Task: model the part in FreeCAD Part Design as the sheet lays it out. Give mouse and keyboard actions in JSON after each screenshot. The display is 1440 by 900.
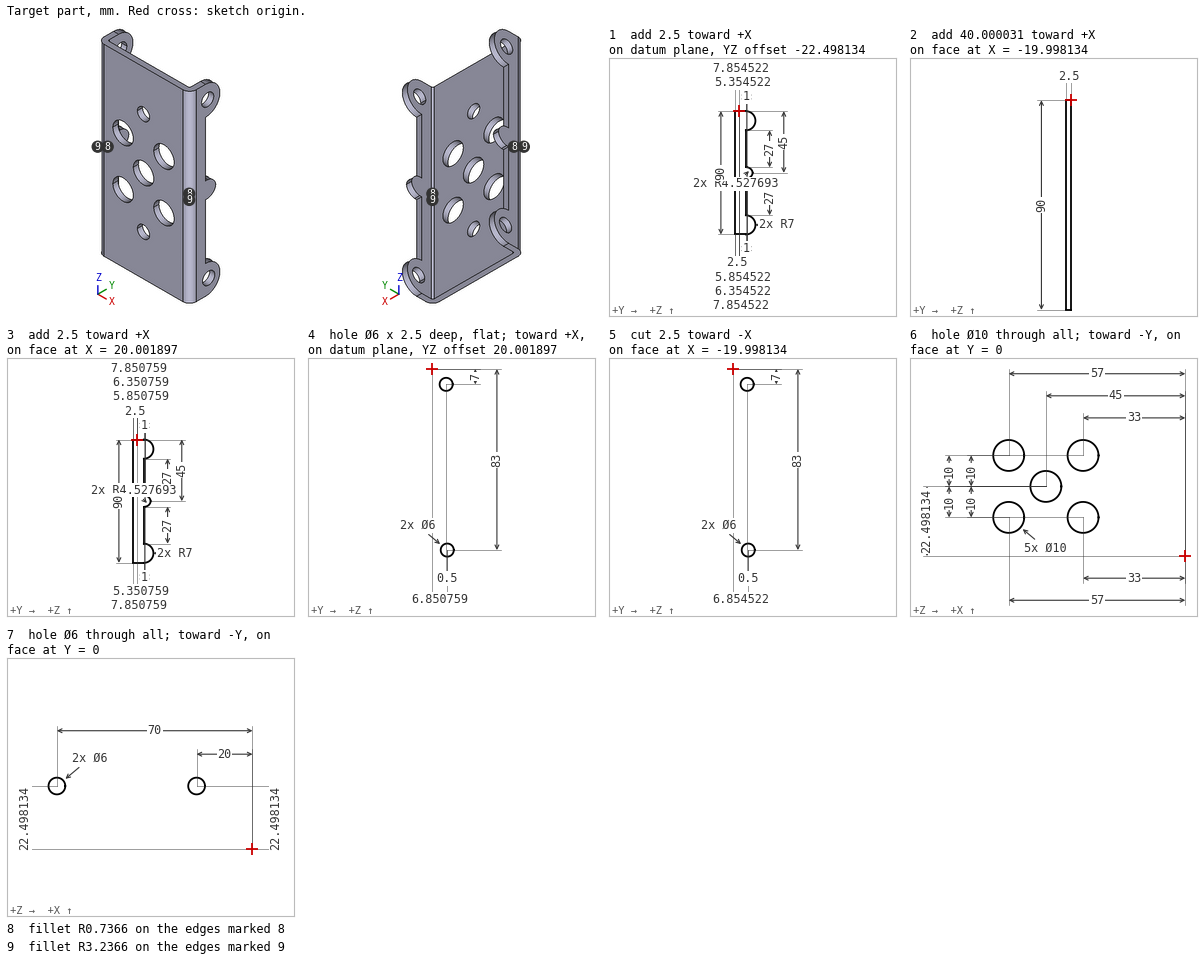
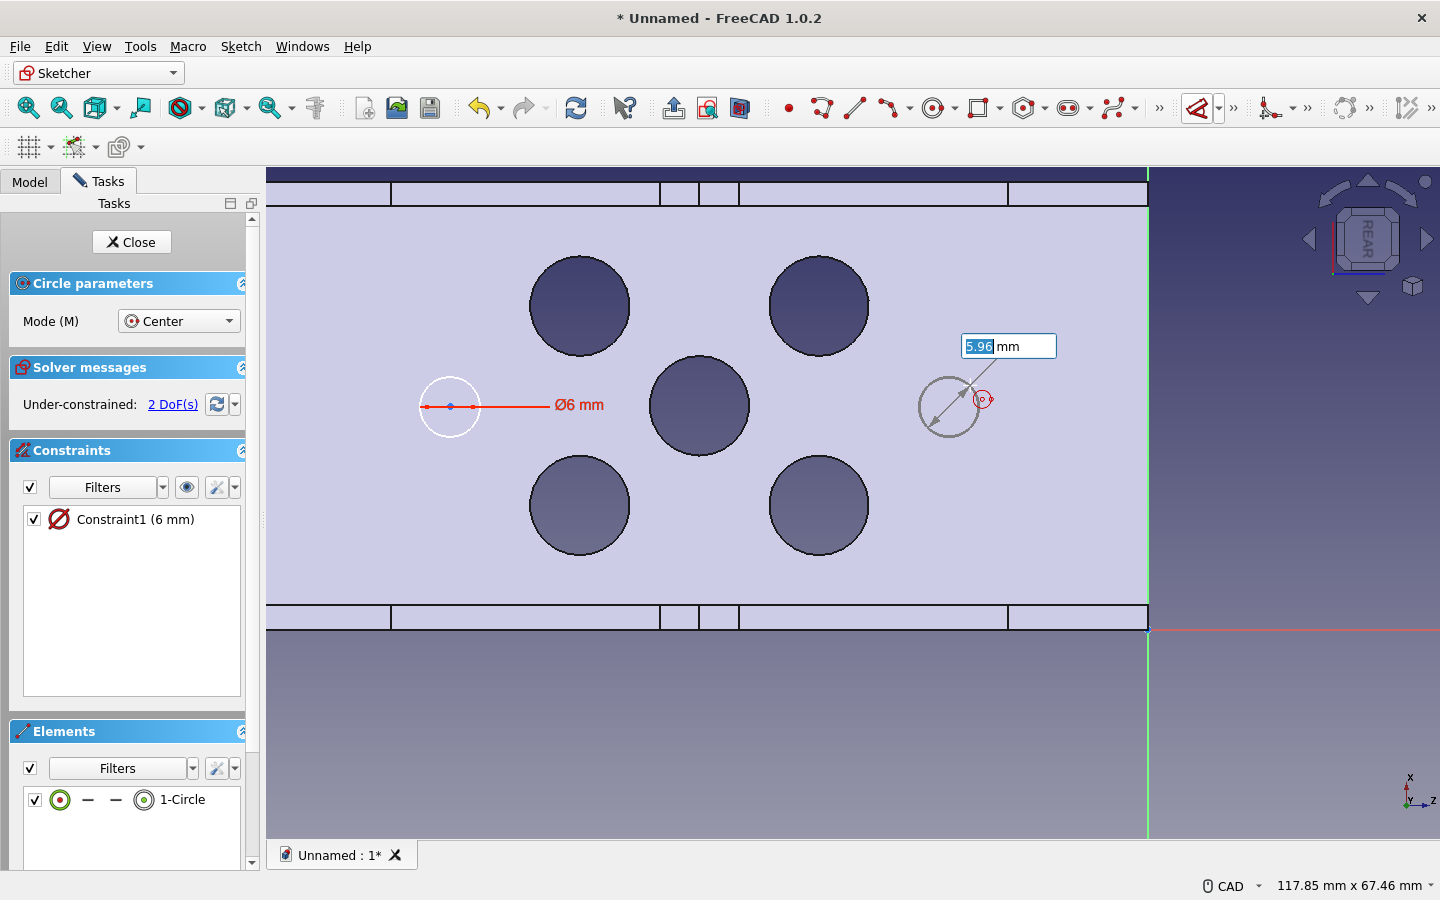
{"action": "type", "text": "6"}
{"action": "key", "text": "Return"}
{"action": "key", "text": "Escape"}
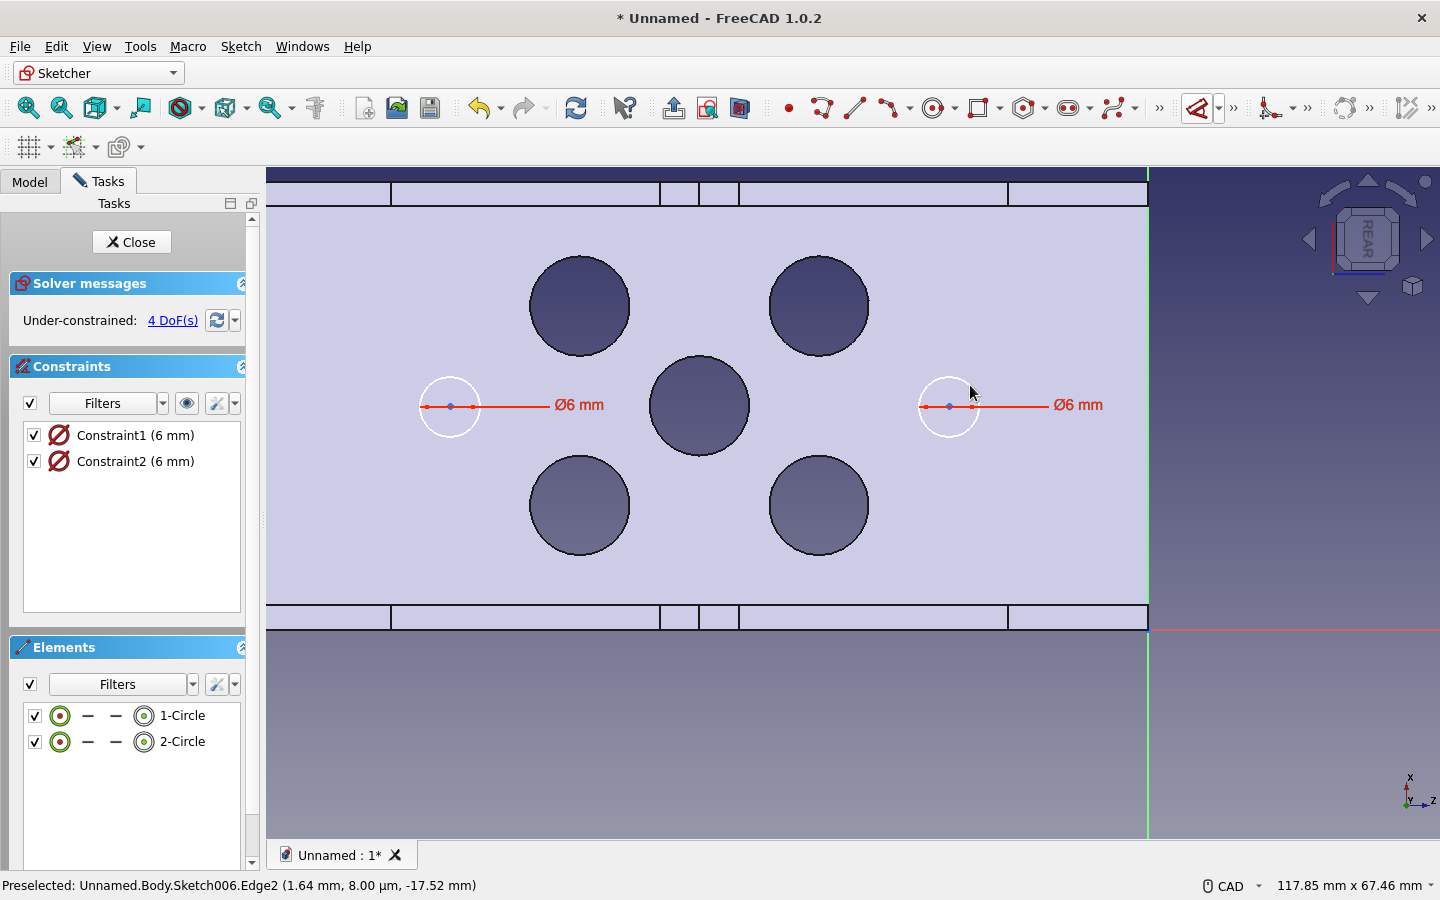
{"action": "left_click", "coordinate": [450, 407]}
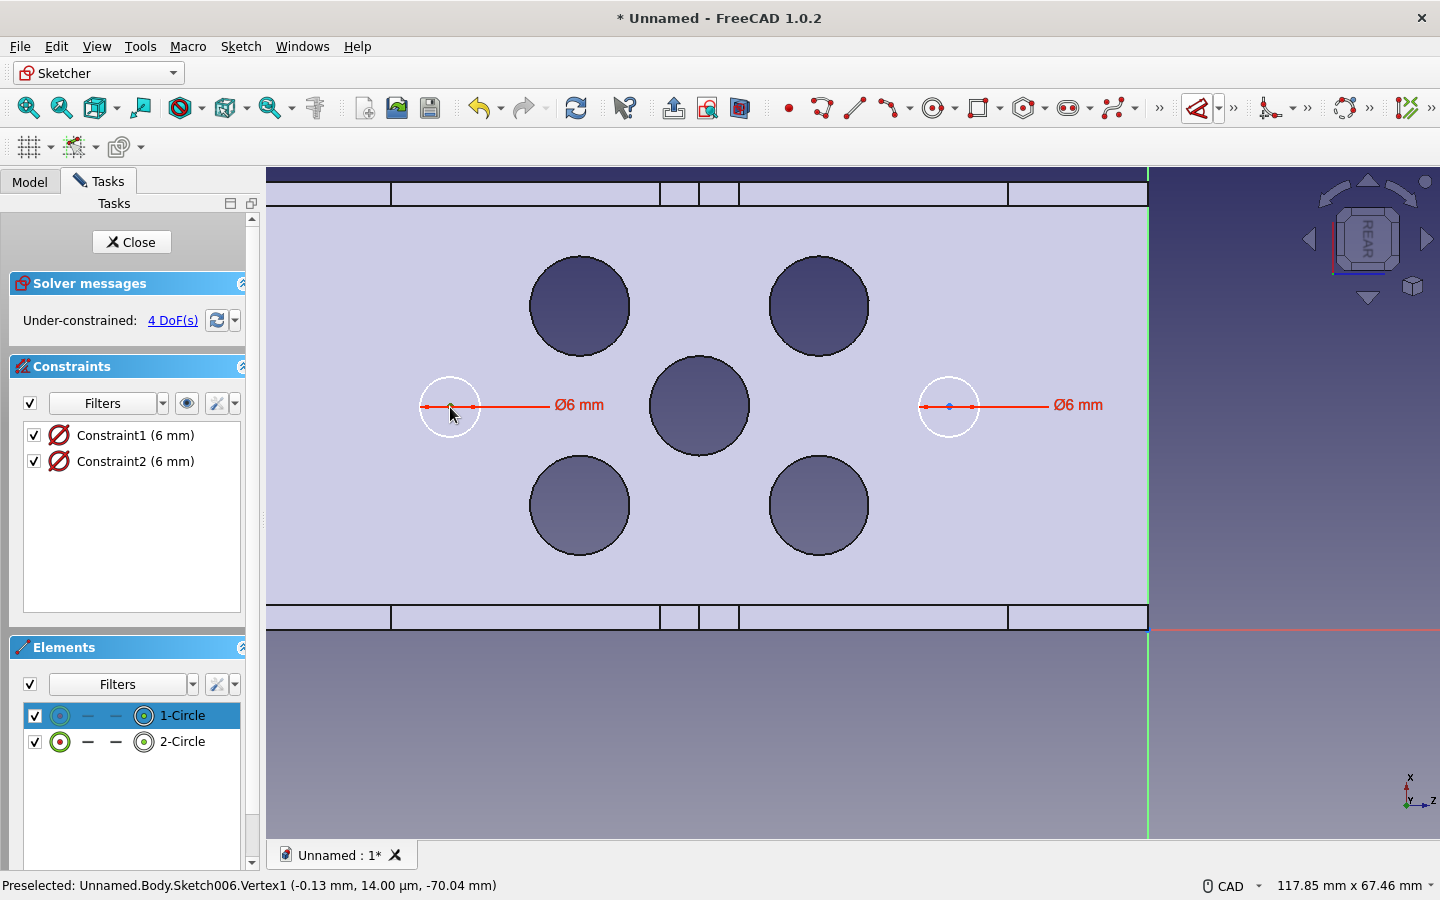
{"action": "left_click", "coordinate": [1218, 108]}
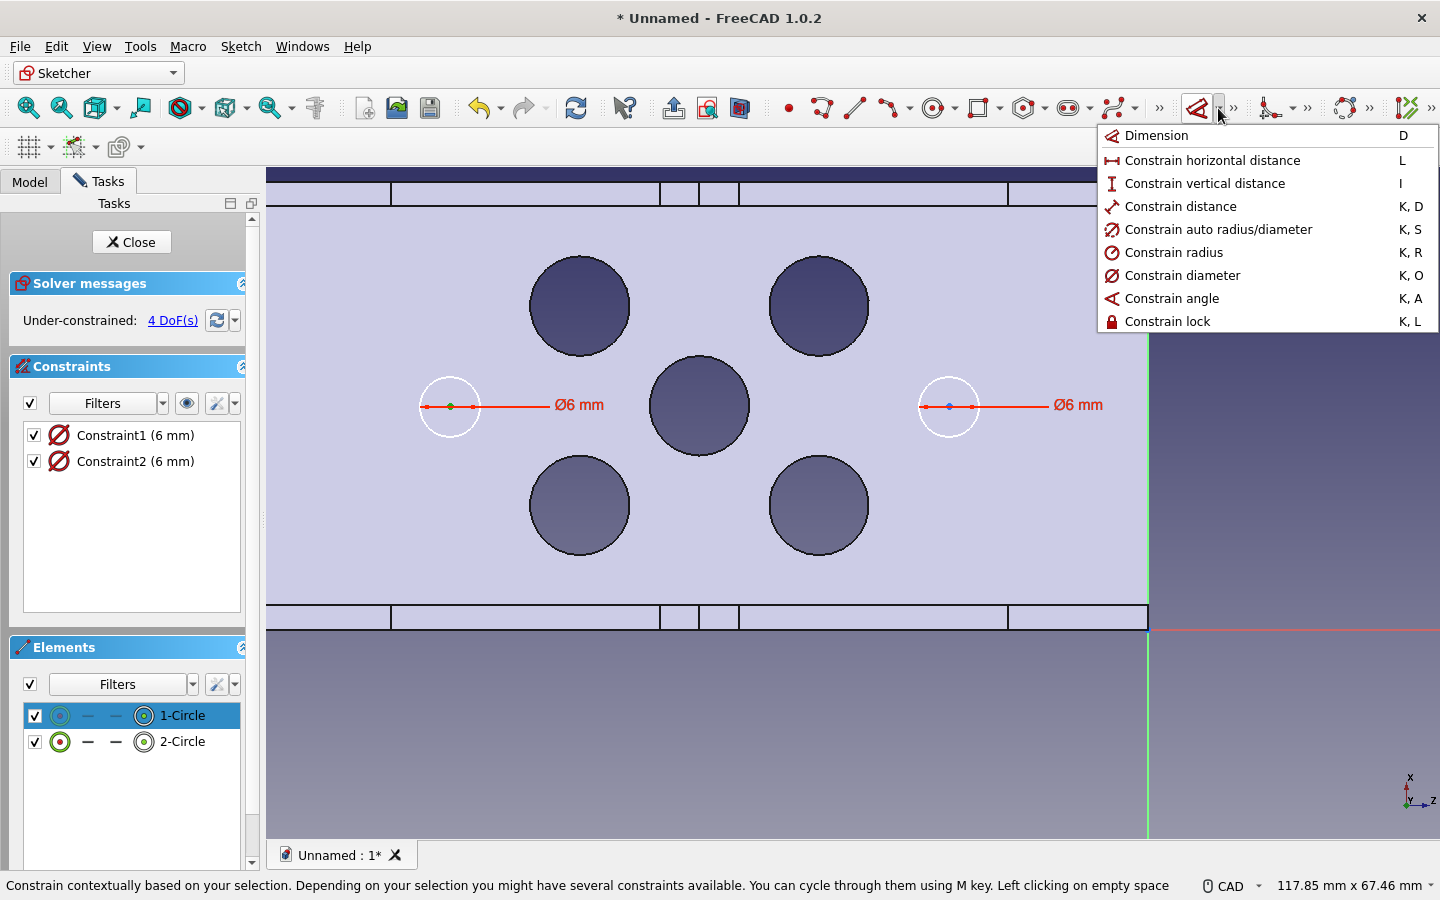
{"action": "left_click", "coordinate": [1268, 160]}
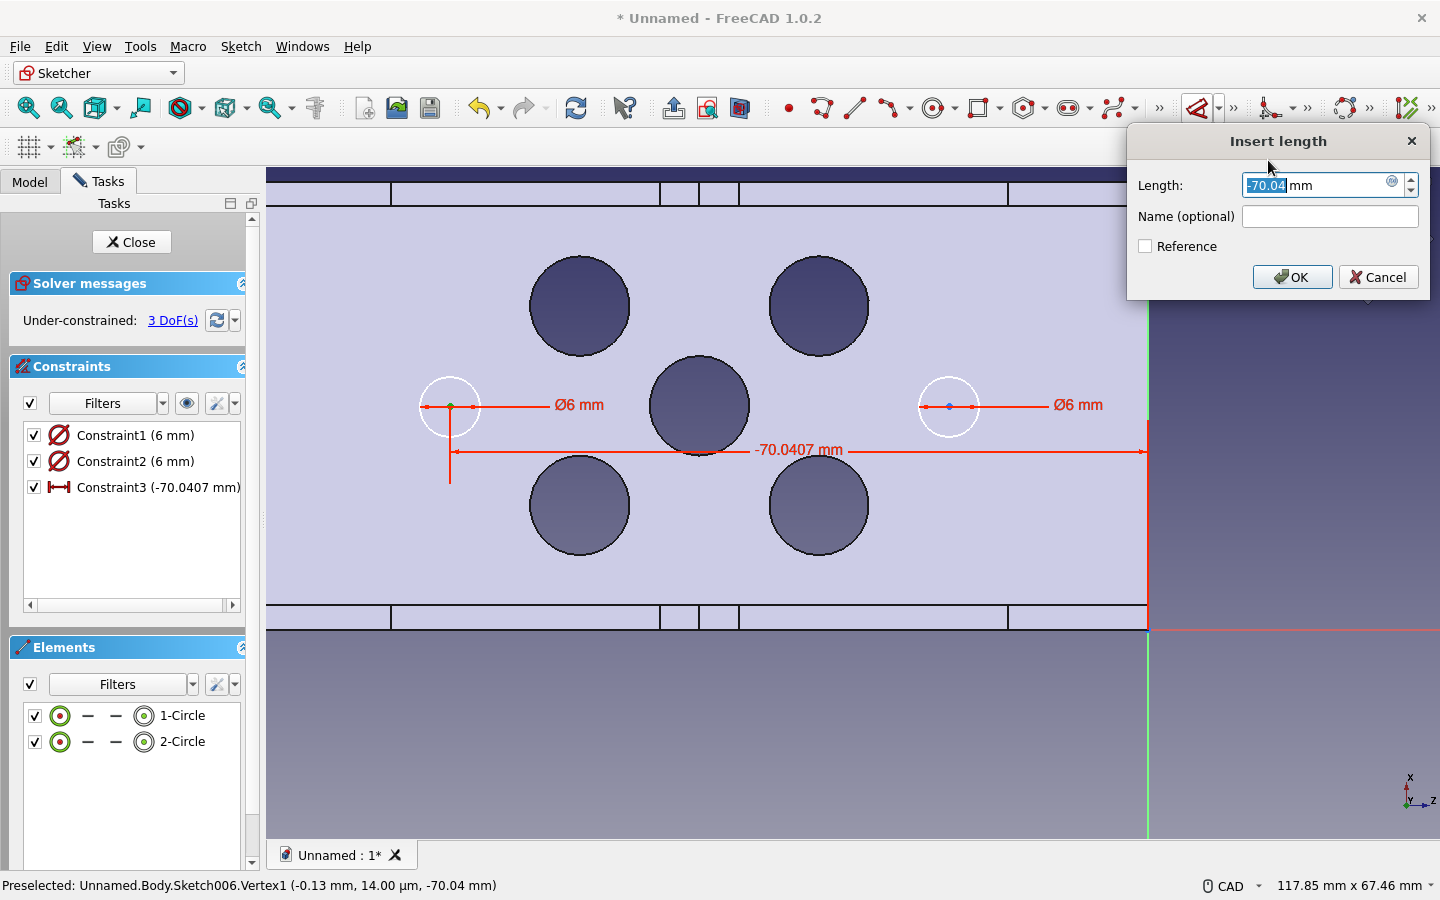
{"action": "type", "text": "-70"}
{"action": "key", "text": "Return"}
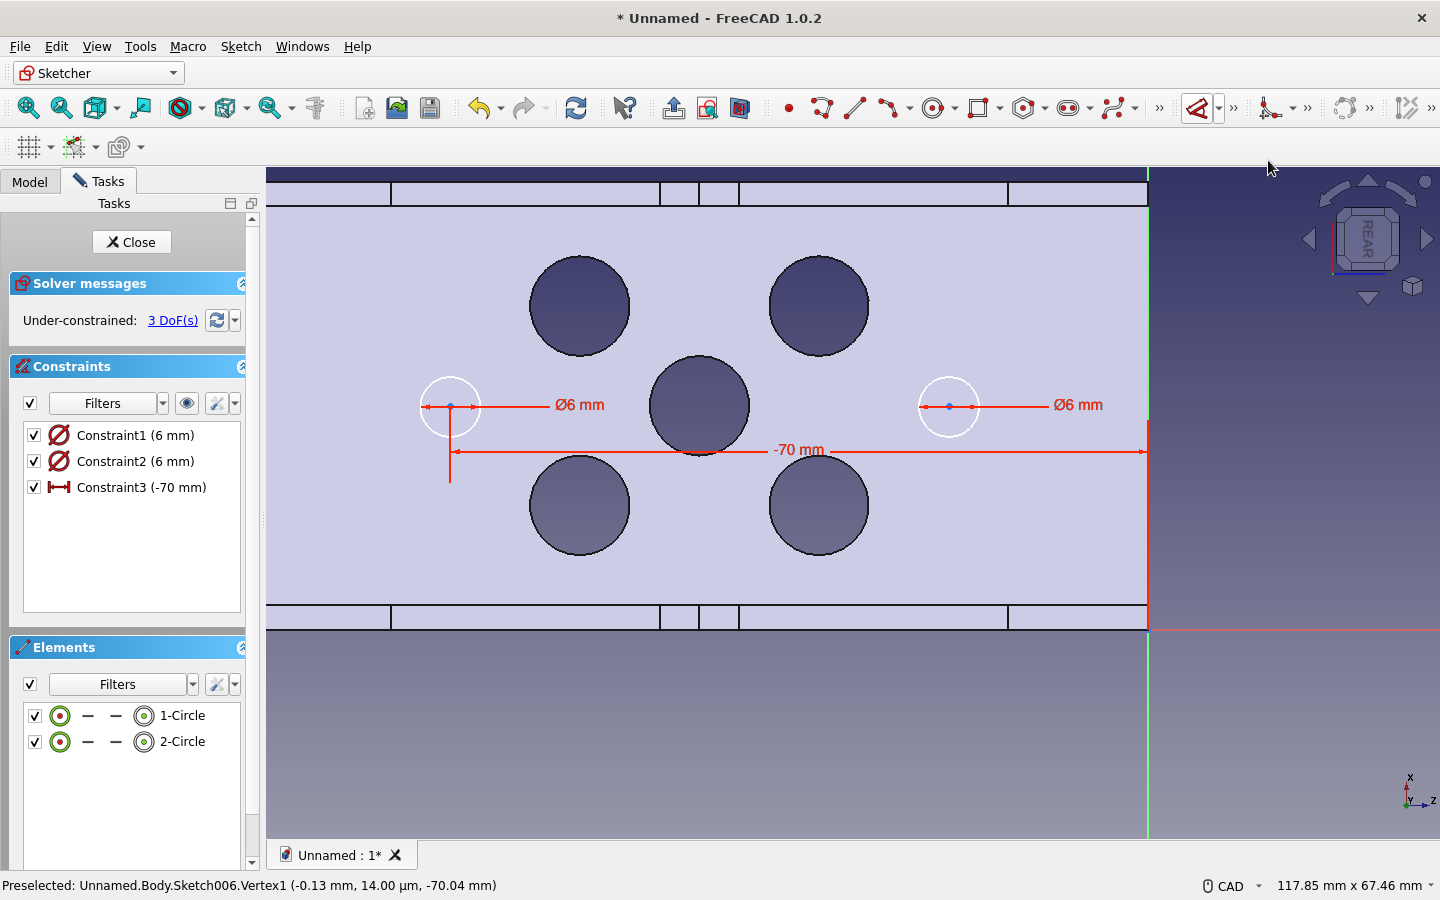
{"action": "left_click", "coordinate": [949, 407]}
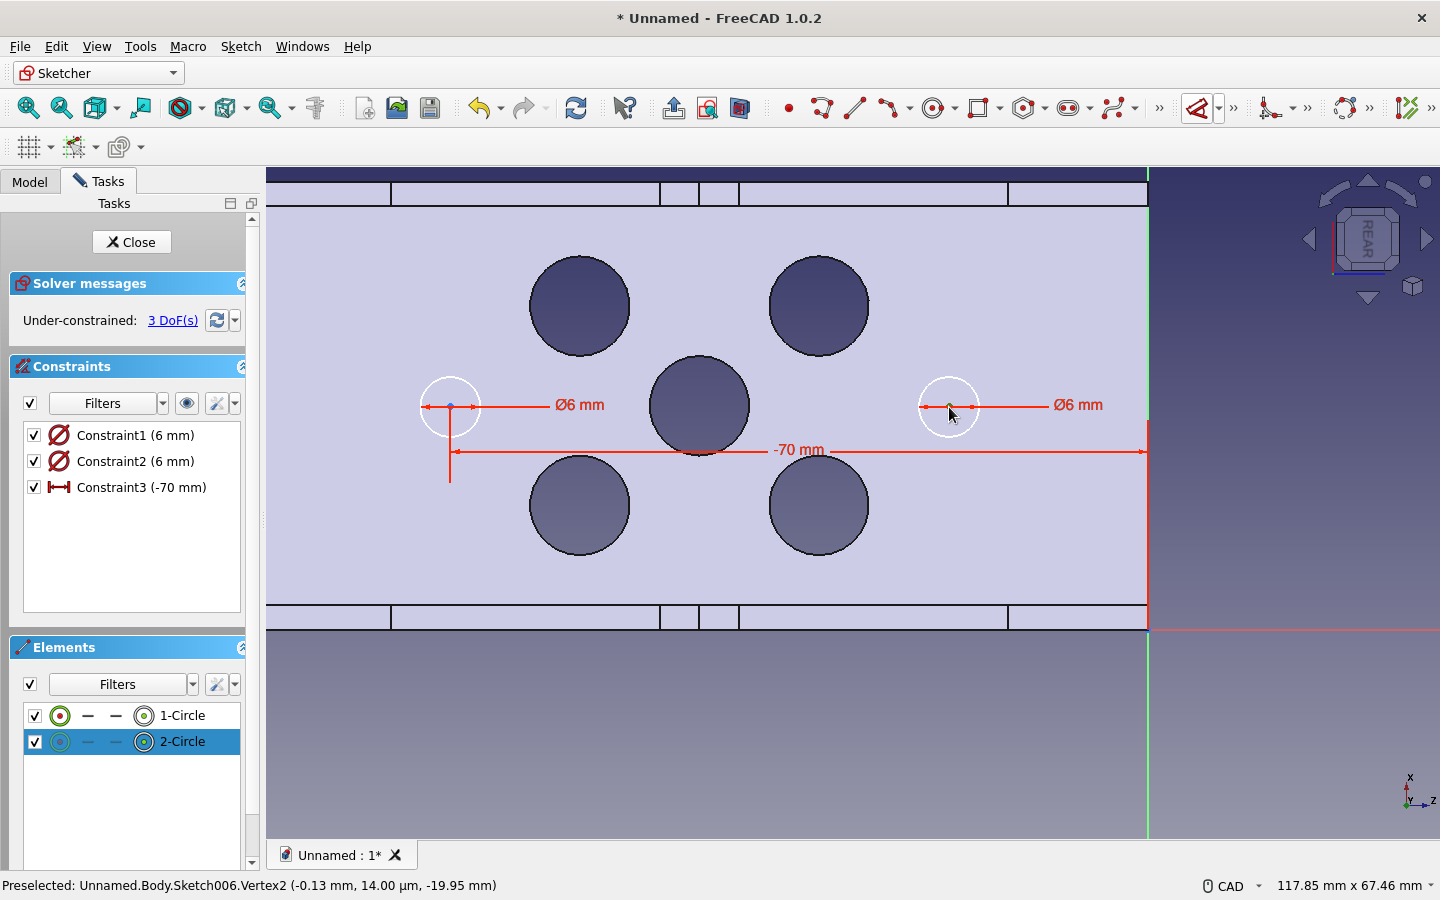
{"action": "key", "text": "l"}